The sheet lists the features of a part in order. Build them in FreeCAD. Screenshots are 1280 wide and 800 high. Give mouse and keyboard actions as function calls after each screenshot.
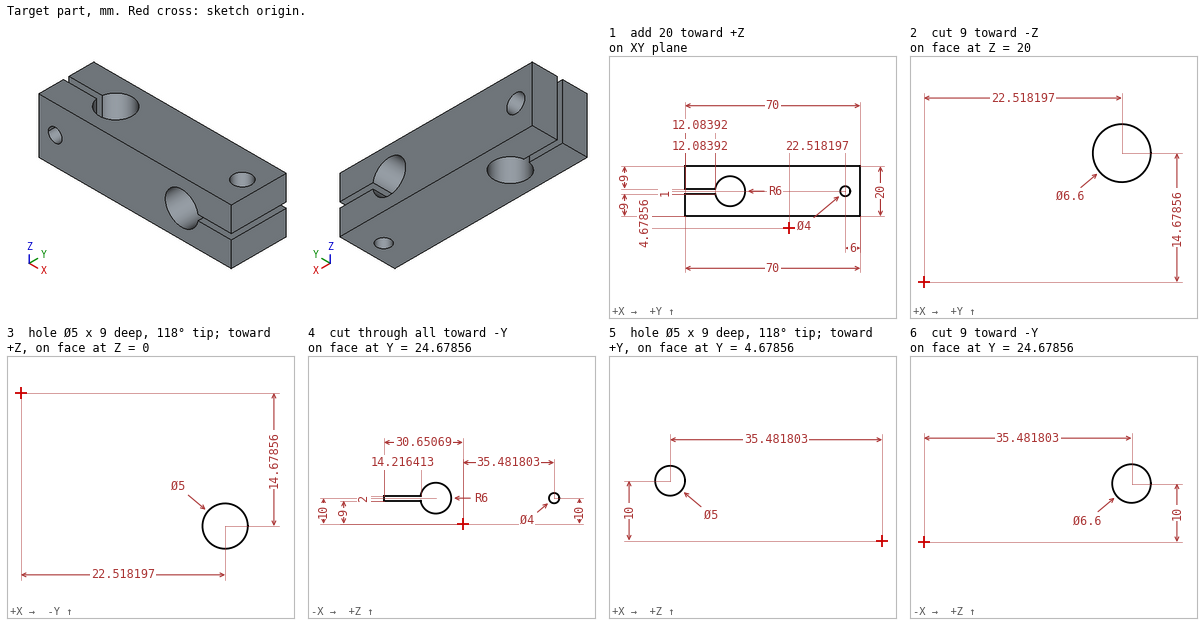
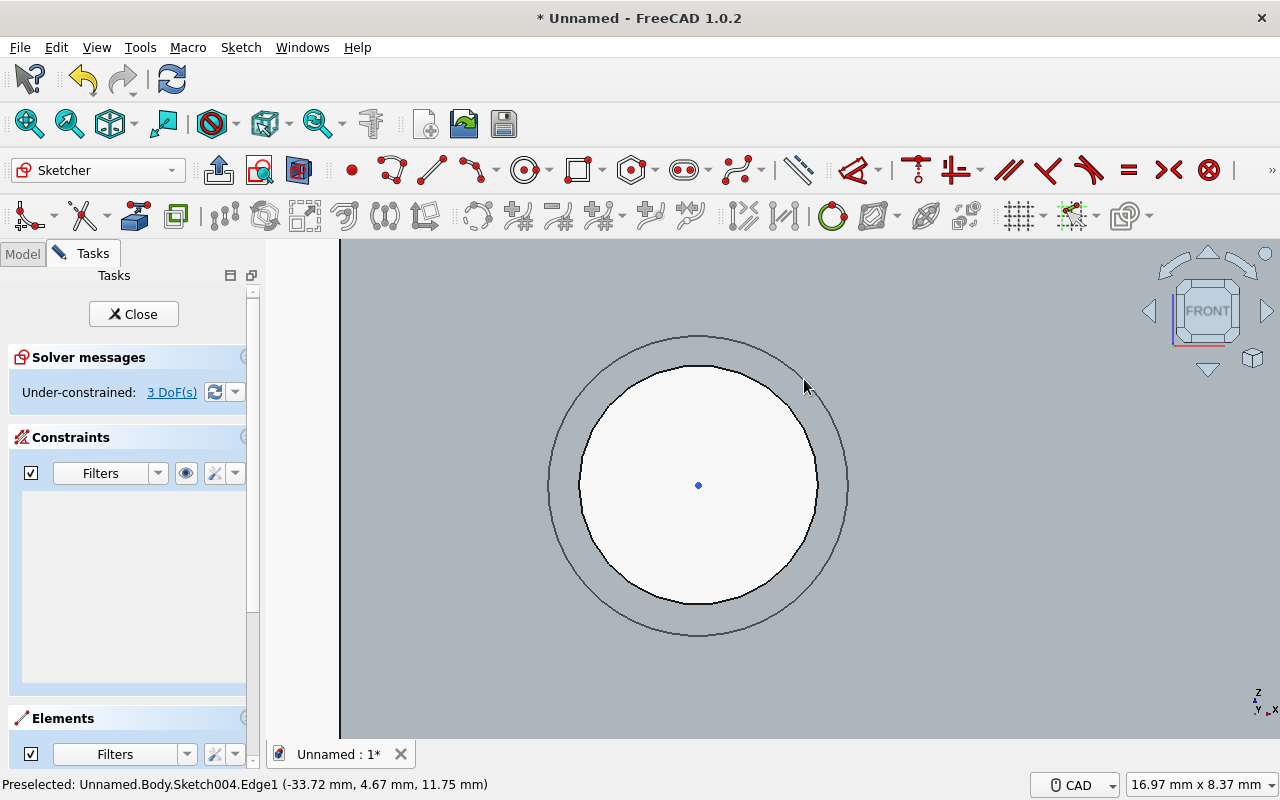
click(854, 170)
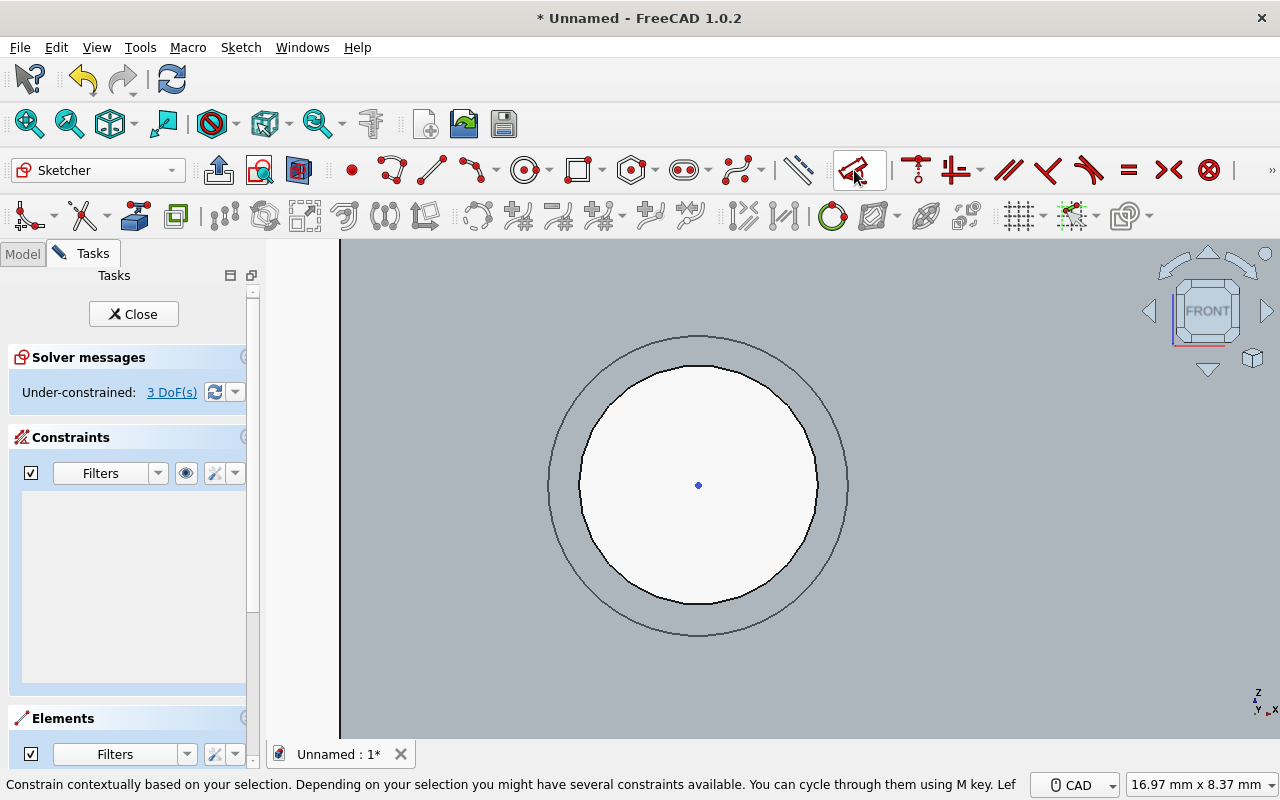
click(804, 380)
click(827, 357)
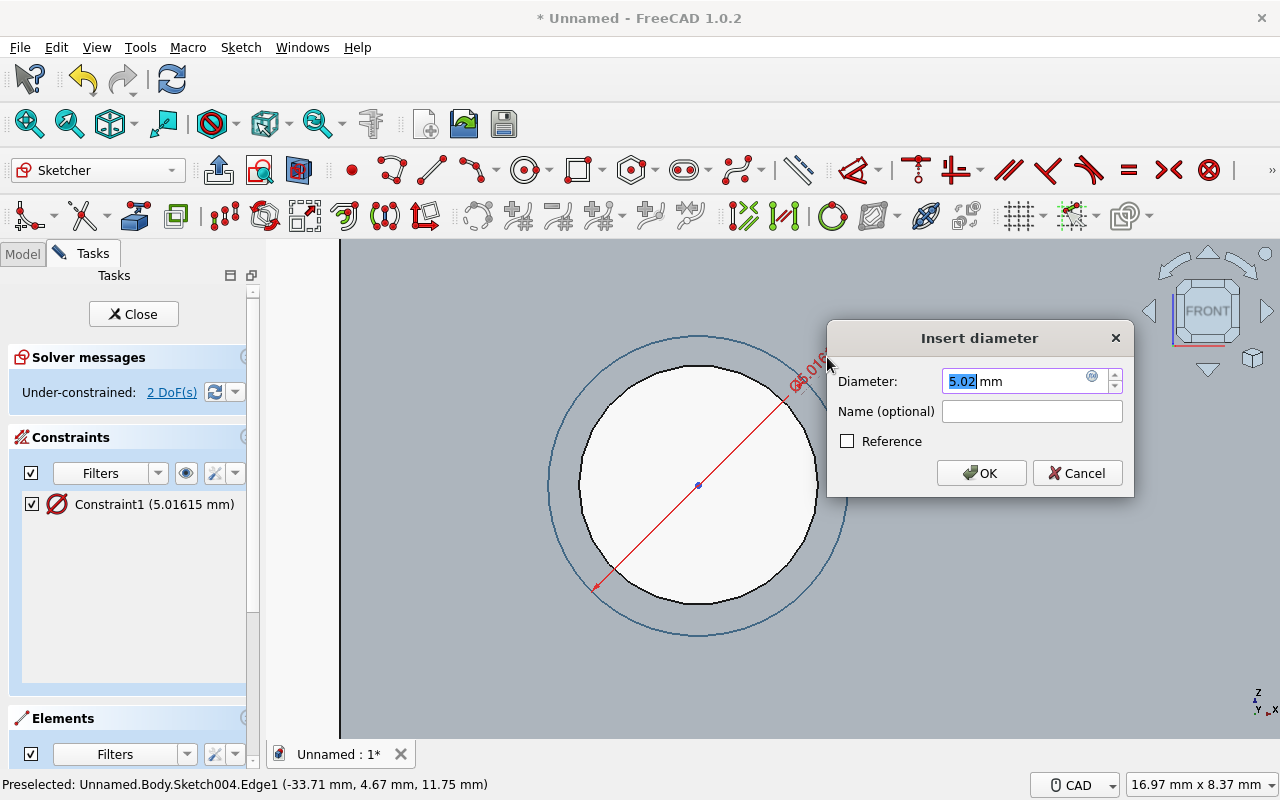
text(5)
key(Return)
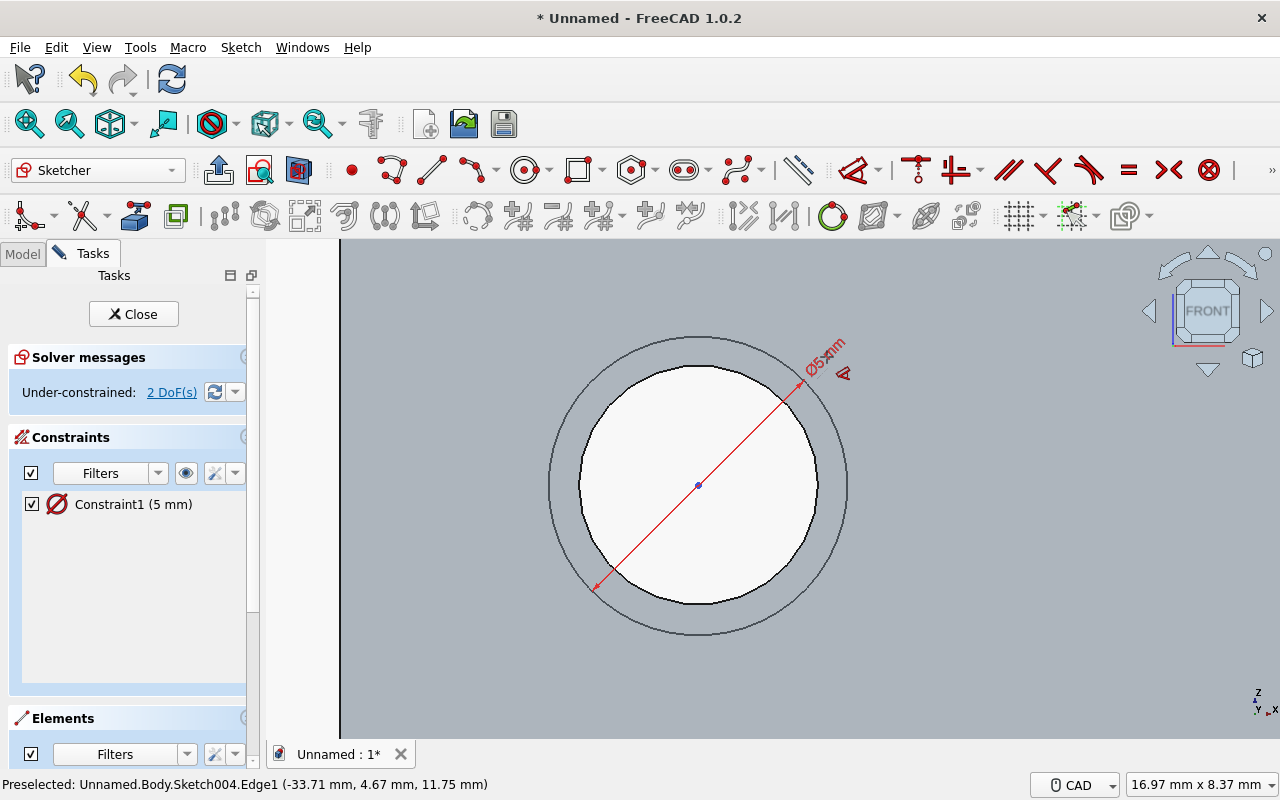
click(698, 486)
click(664, 599)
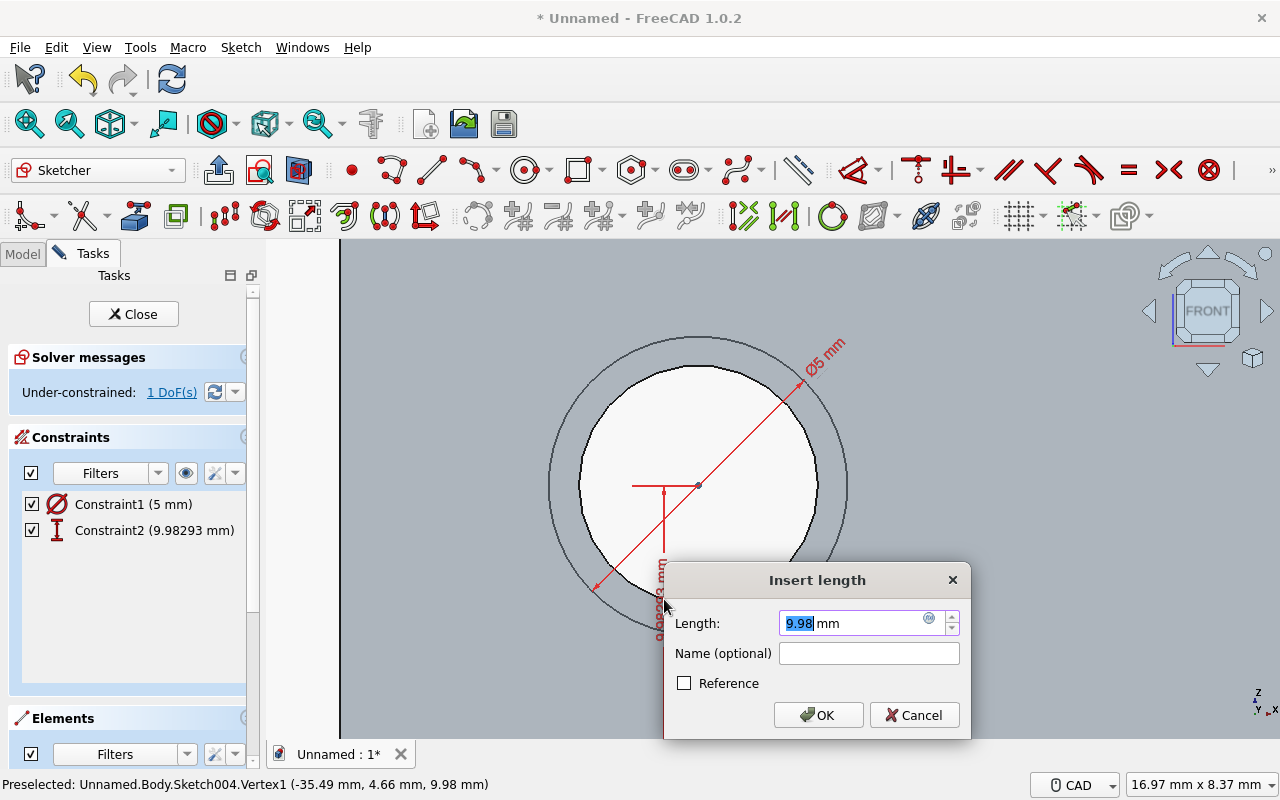
text(10)
key(Return)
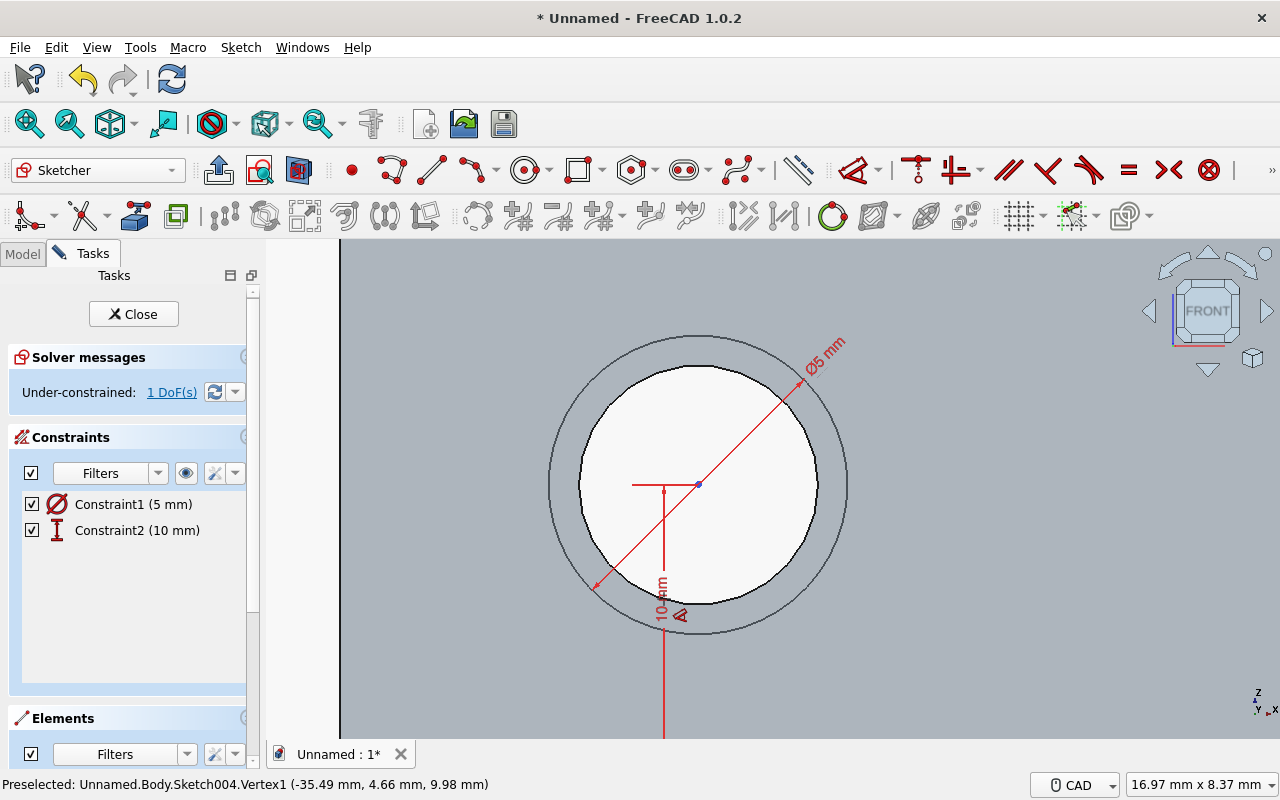
click(698, 485)
click(907, 451)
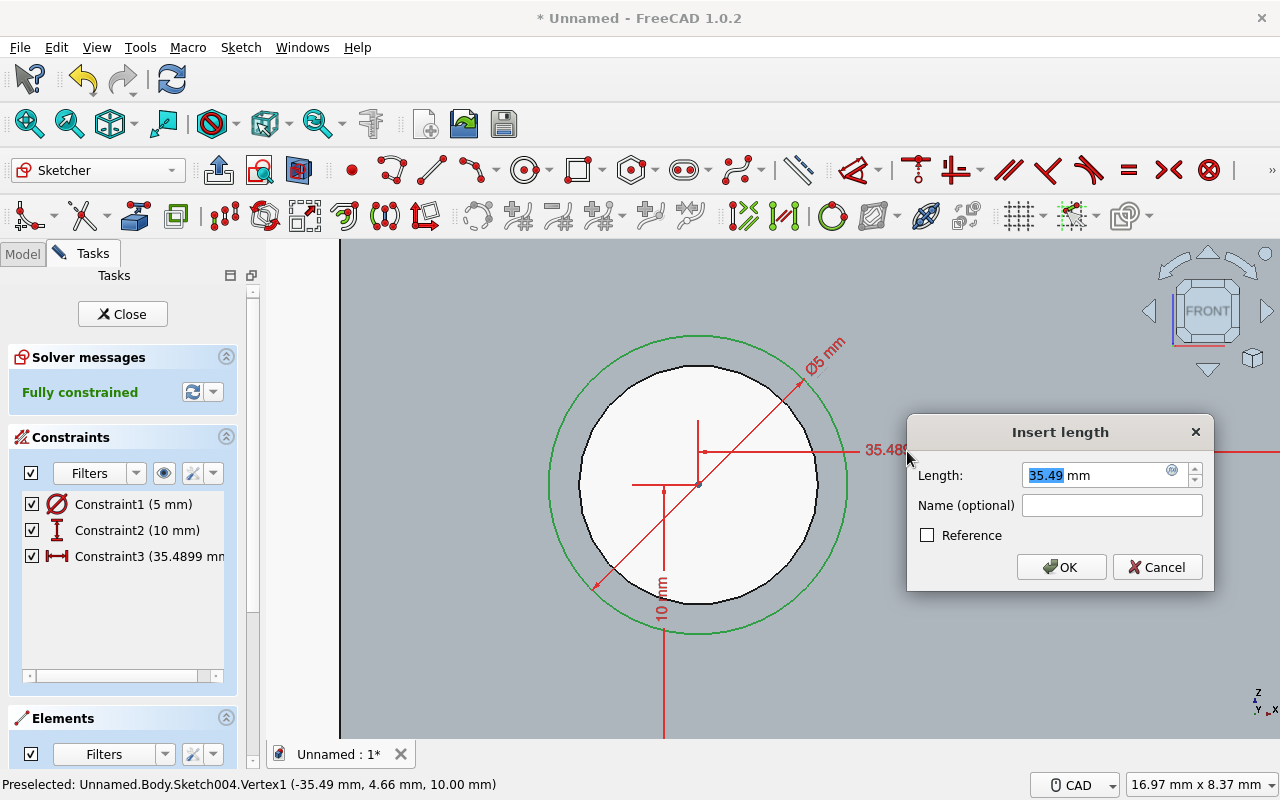
text(35.481803)
key(Return)
key(Escape)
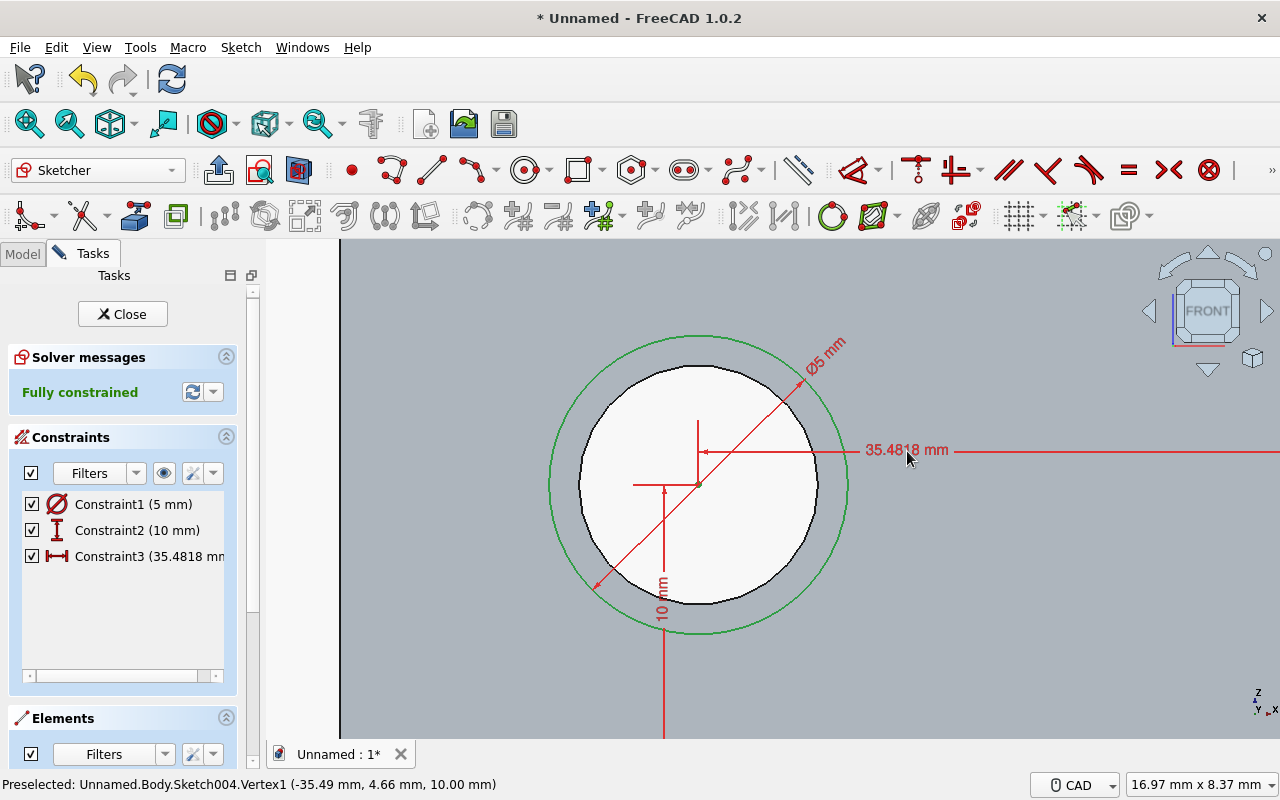
click(123, 314)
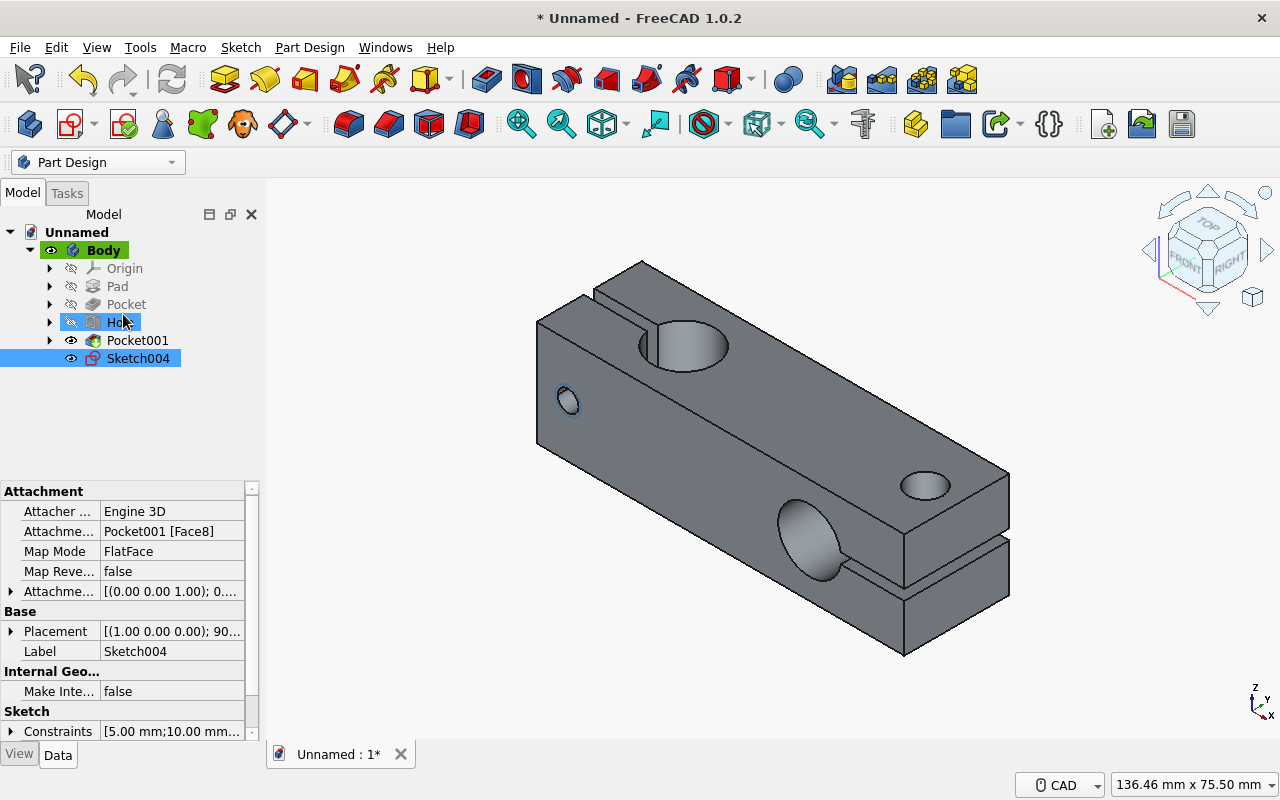
click(528, 80)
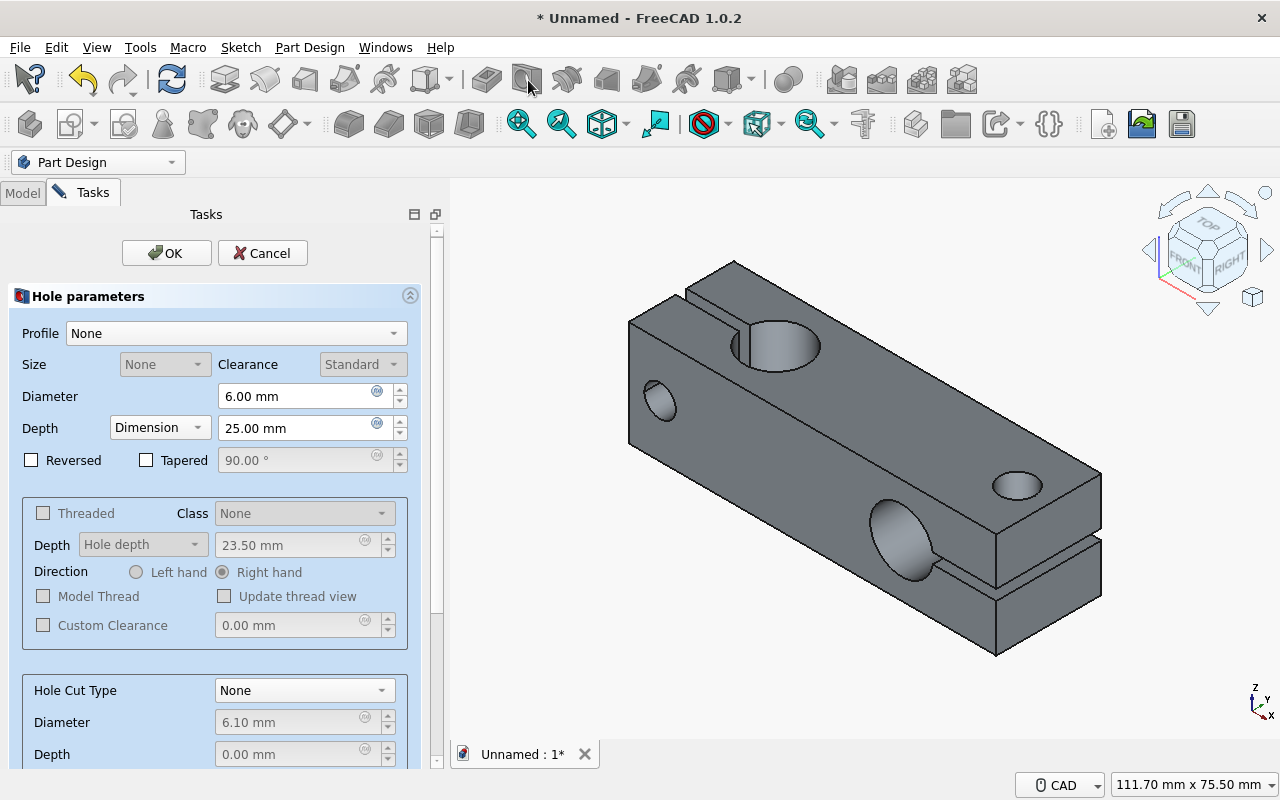
triple_click(305, 396)